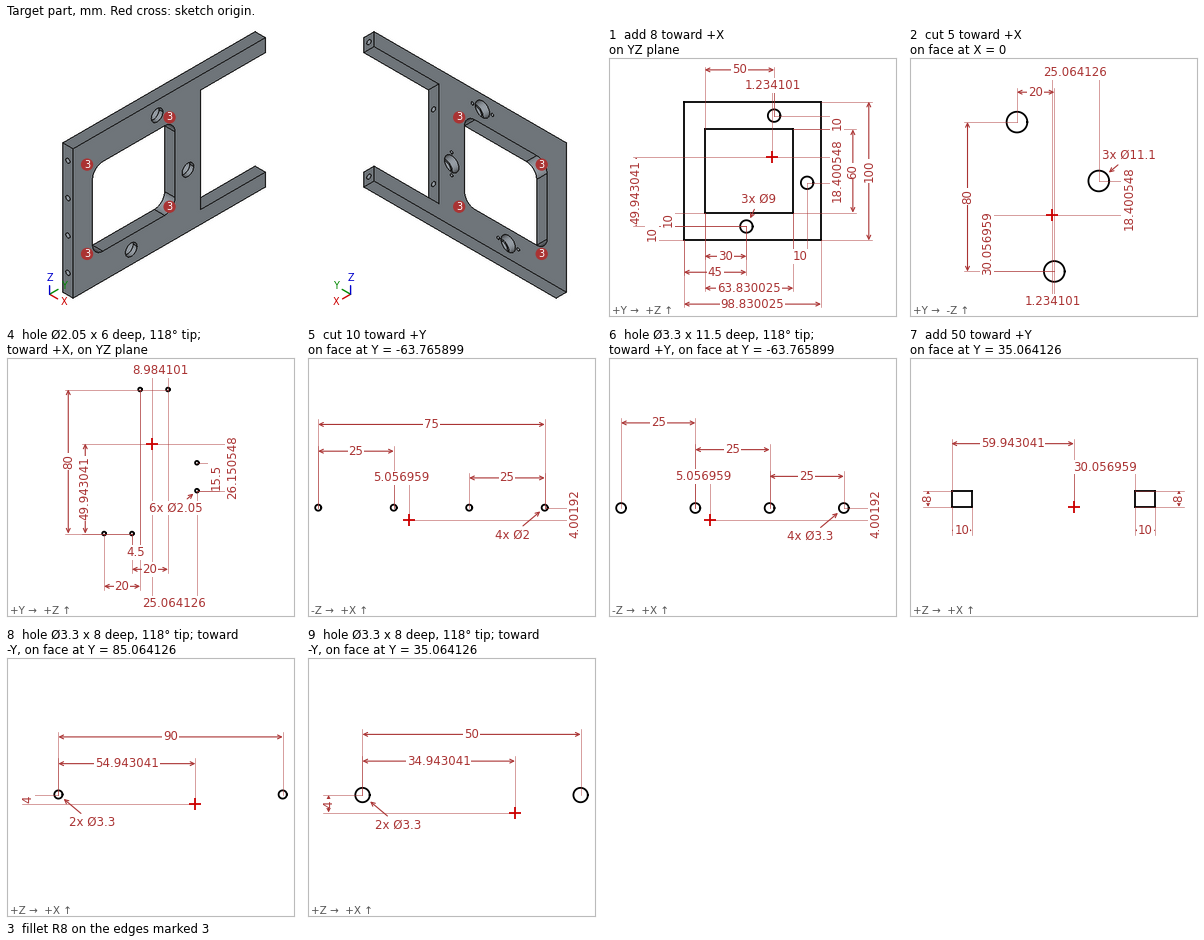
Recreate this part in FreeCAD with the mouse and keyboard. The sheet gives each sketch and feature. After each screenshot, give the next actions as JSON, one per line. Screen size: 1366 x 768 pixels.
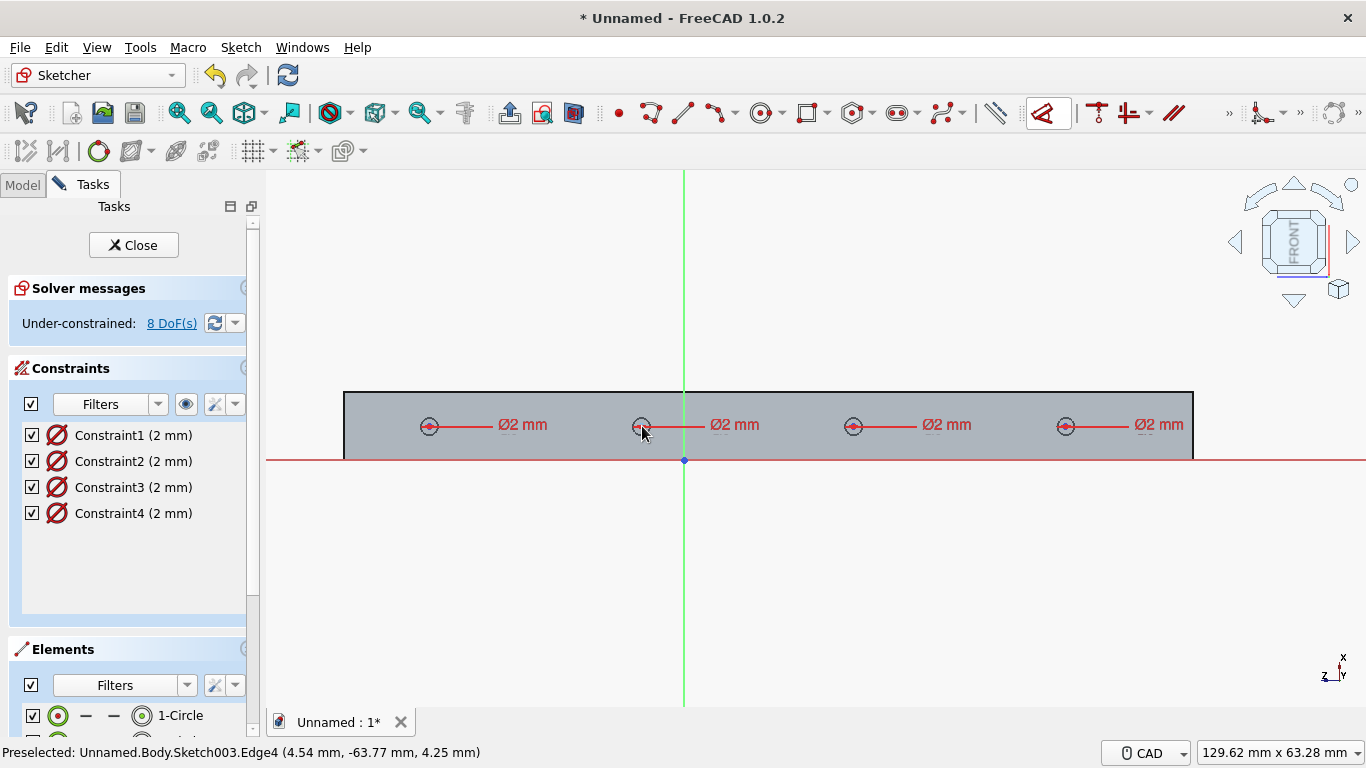
{"action": "left_click", "coordinate": [1066, 427]}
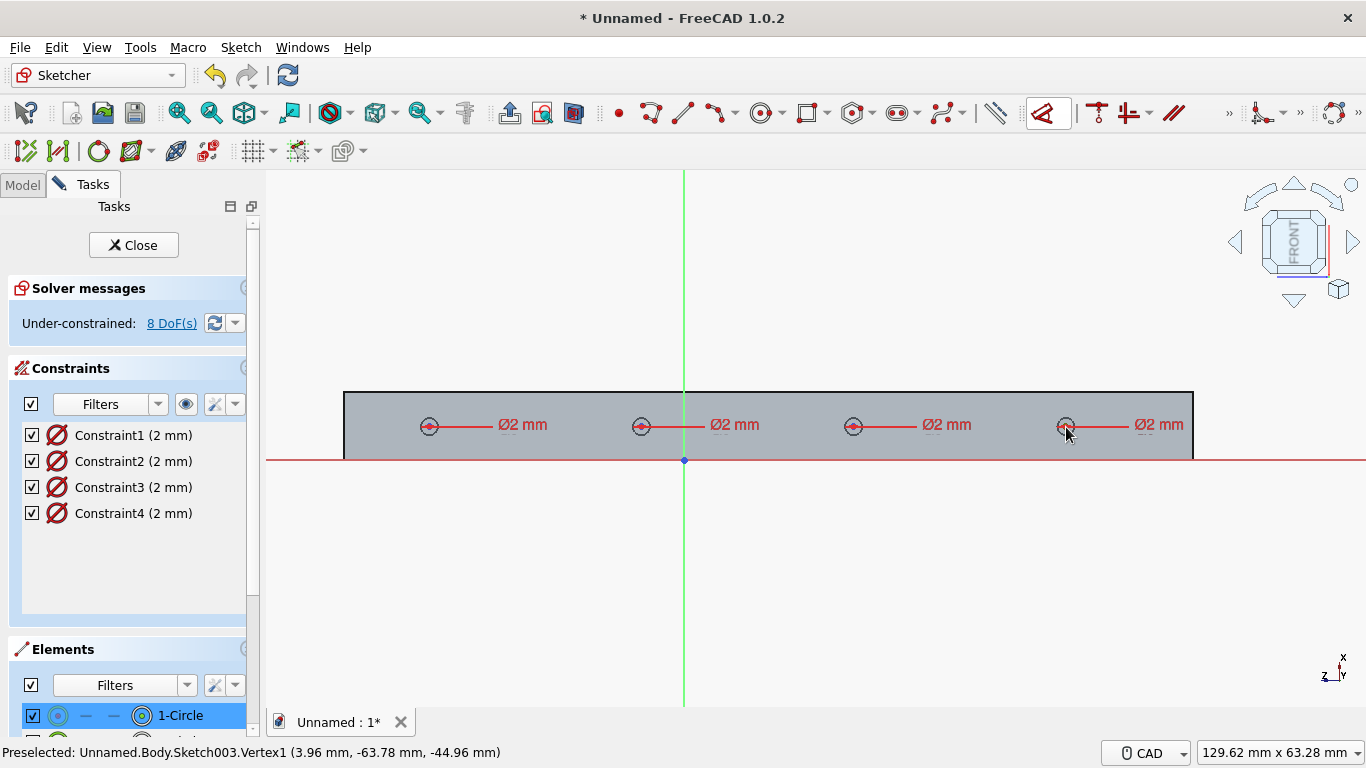
{"action": "left_click", "coordinate": [429, 427]}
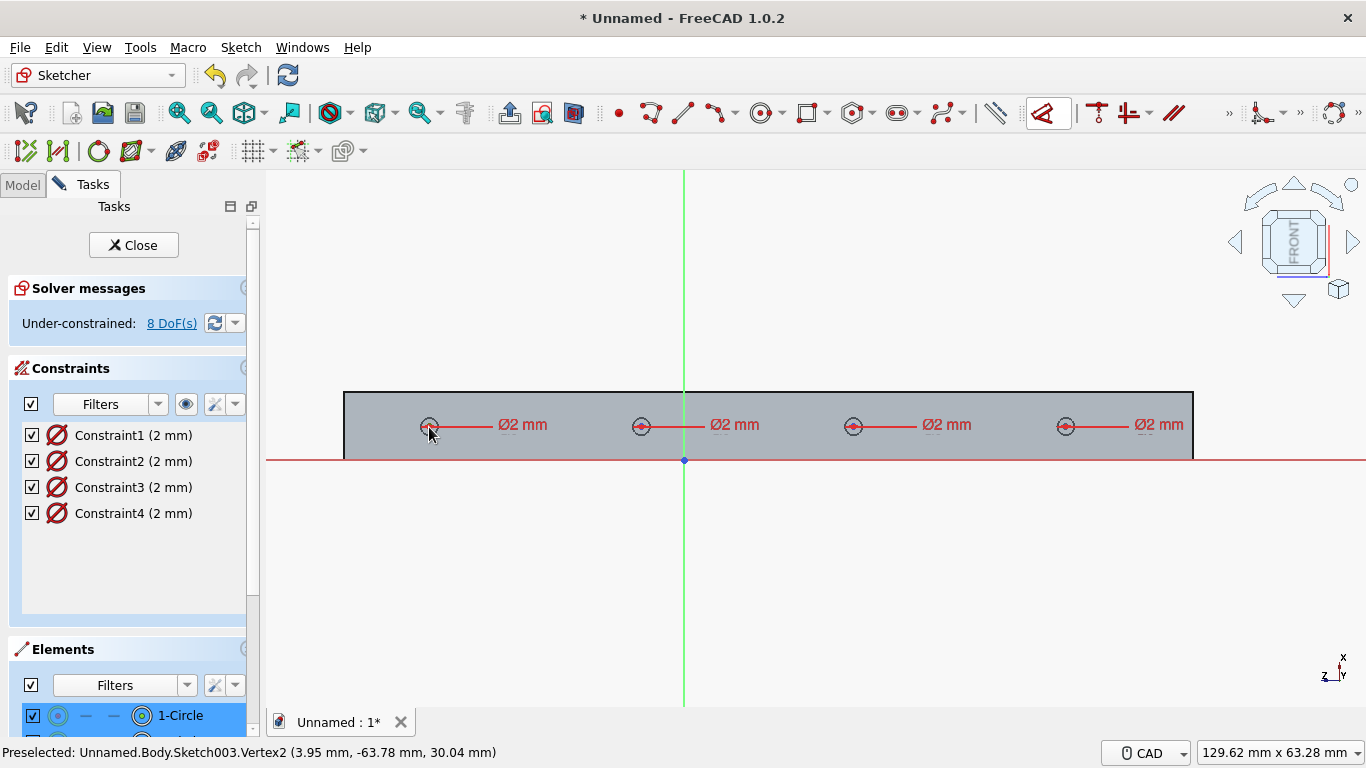
{"action": "key", "text": "h"}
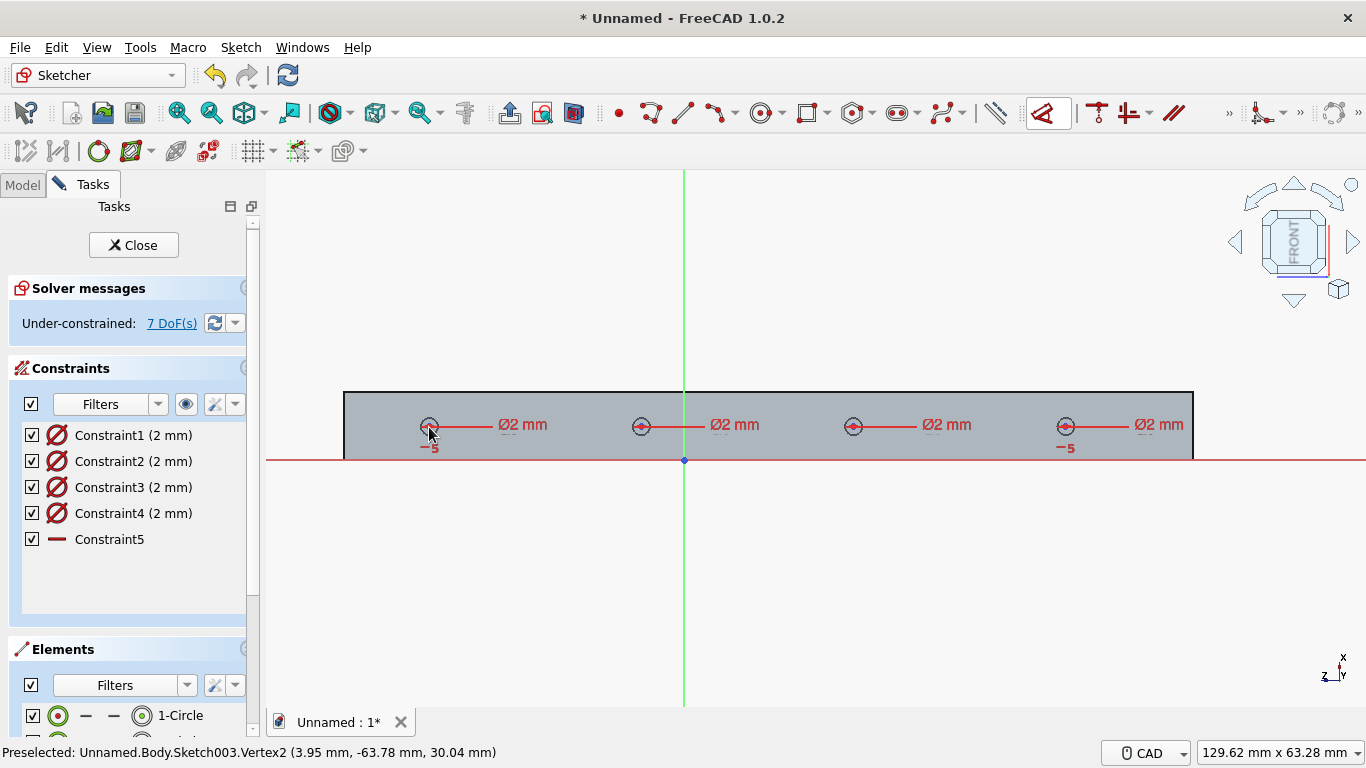
{"action": "left_click", "coordinate": [1066, 427]}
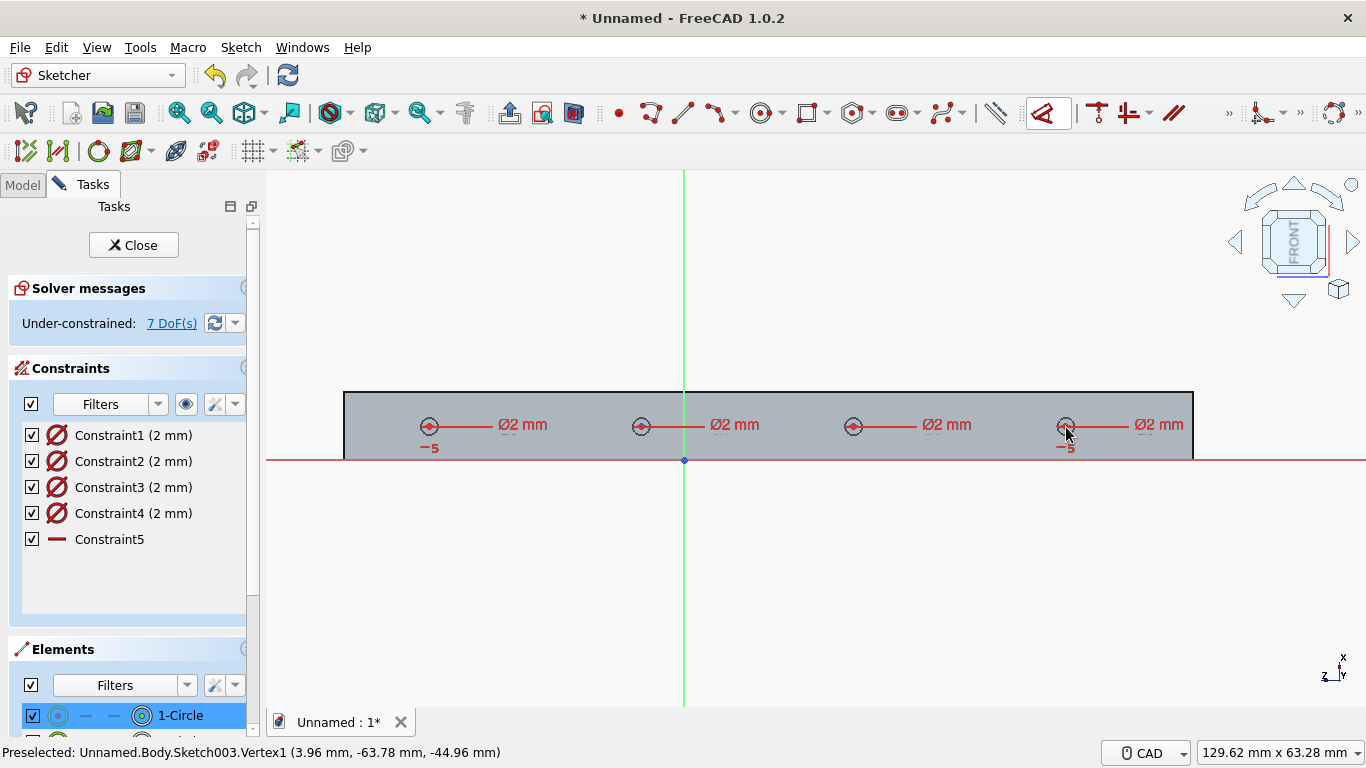
{"action": "left_click", "coordinate": [854, 427]}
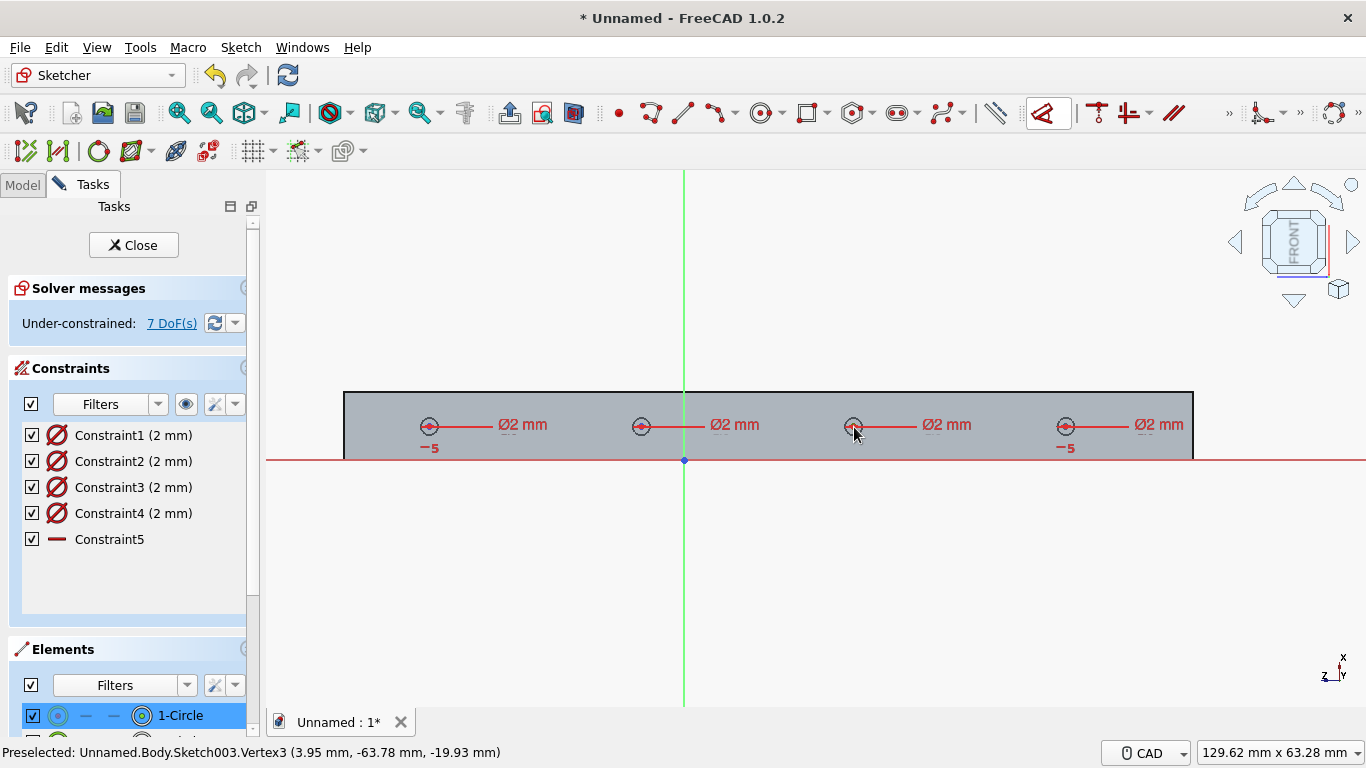
{"action": "left_click", "coordinate": [1152, 114]}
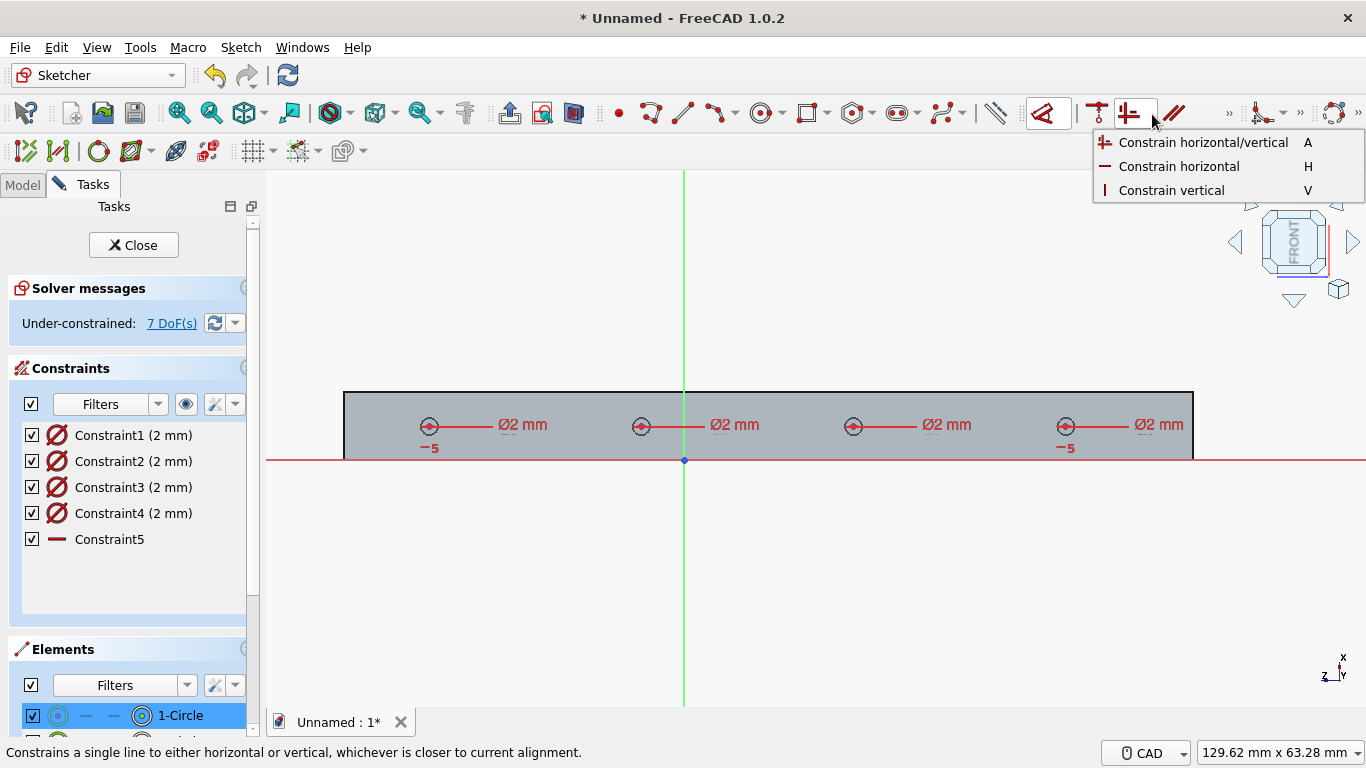
{"action": "left_click", "coordinate": [1229, 166]}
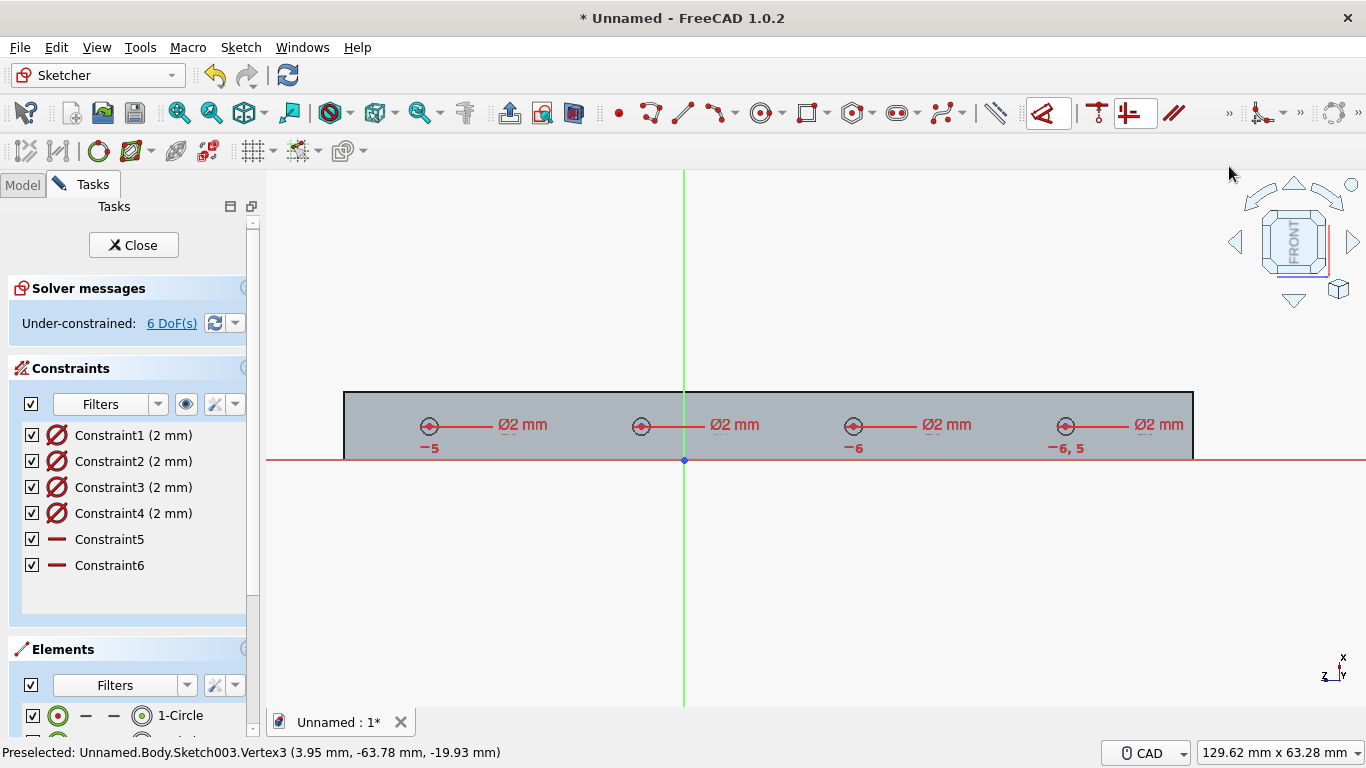
{"action": "left_click", "coordinate": [429, 427]}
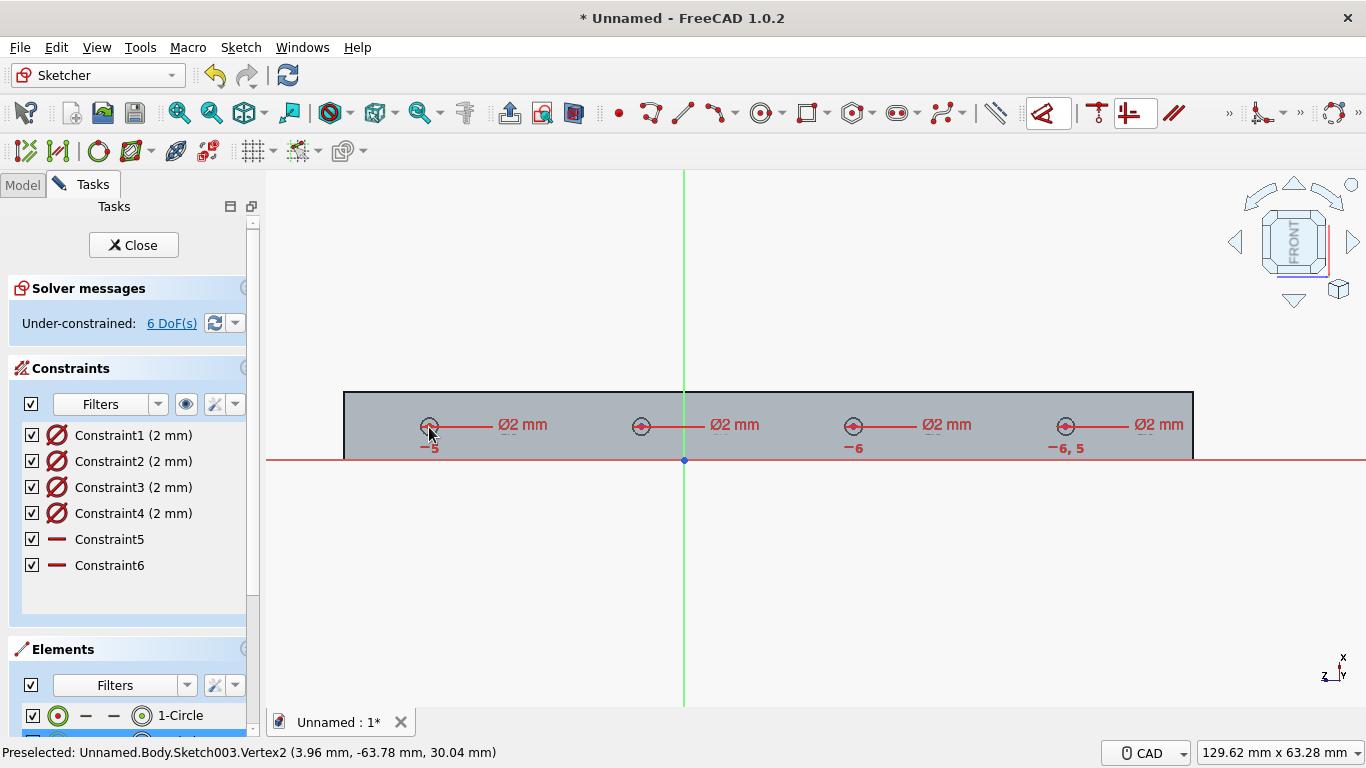
{"action": "left_click", "coordinate": [641, 427]}